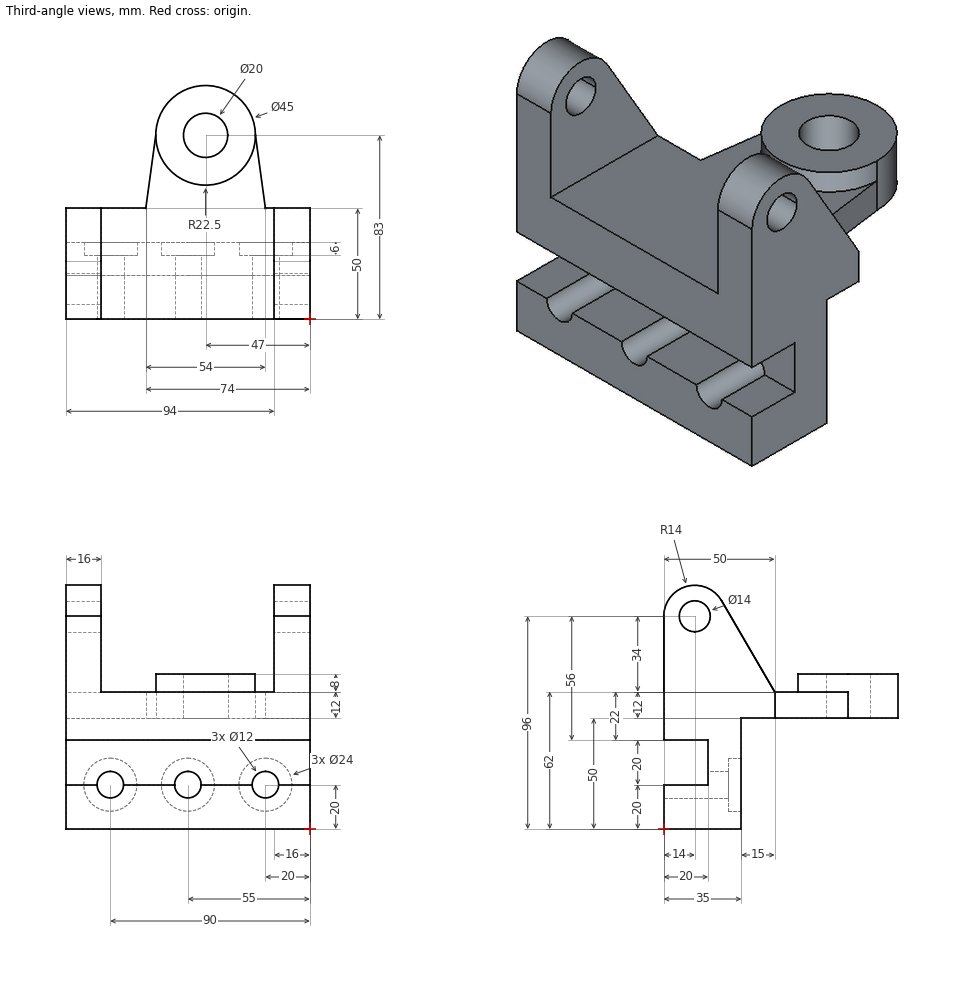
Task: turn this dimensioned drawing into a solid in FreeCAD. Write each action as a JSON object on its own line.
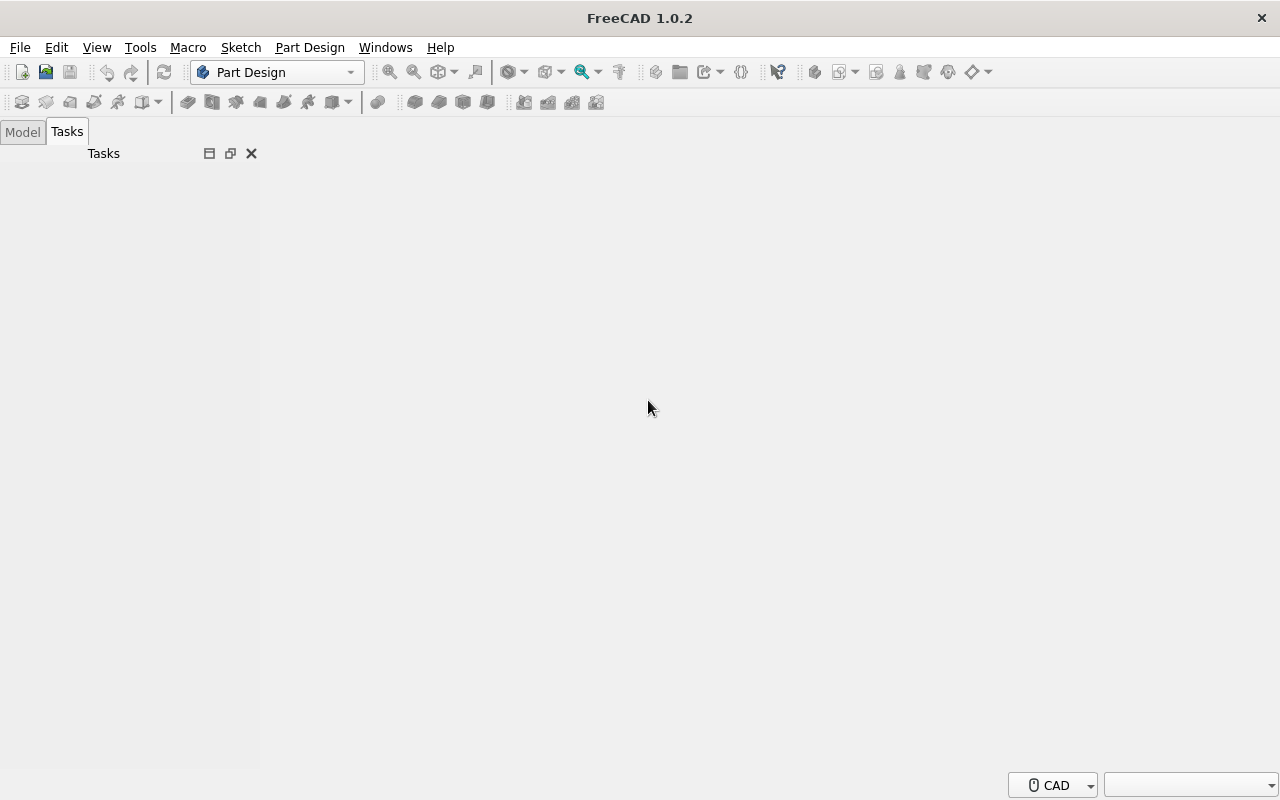
{"action": "key", "text": "ctrl+n"}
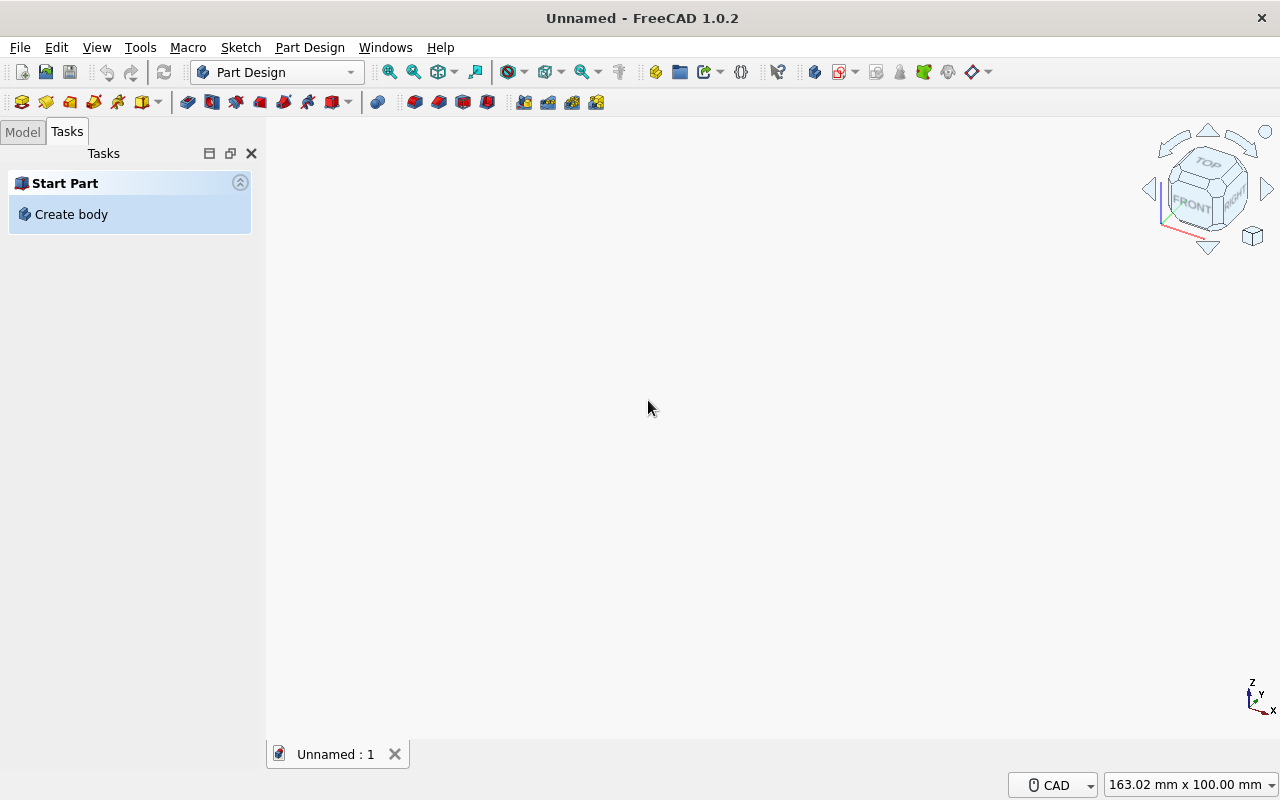
{"action": "left_click", "coordinate": [840, 72]}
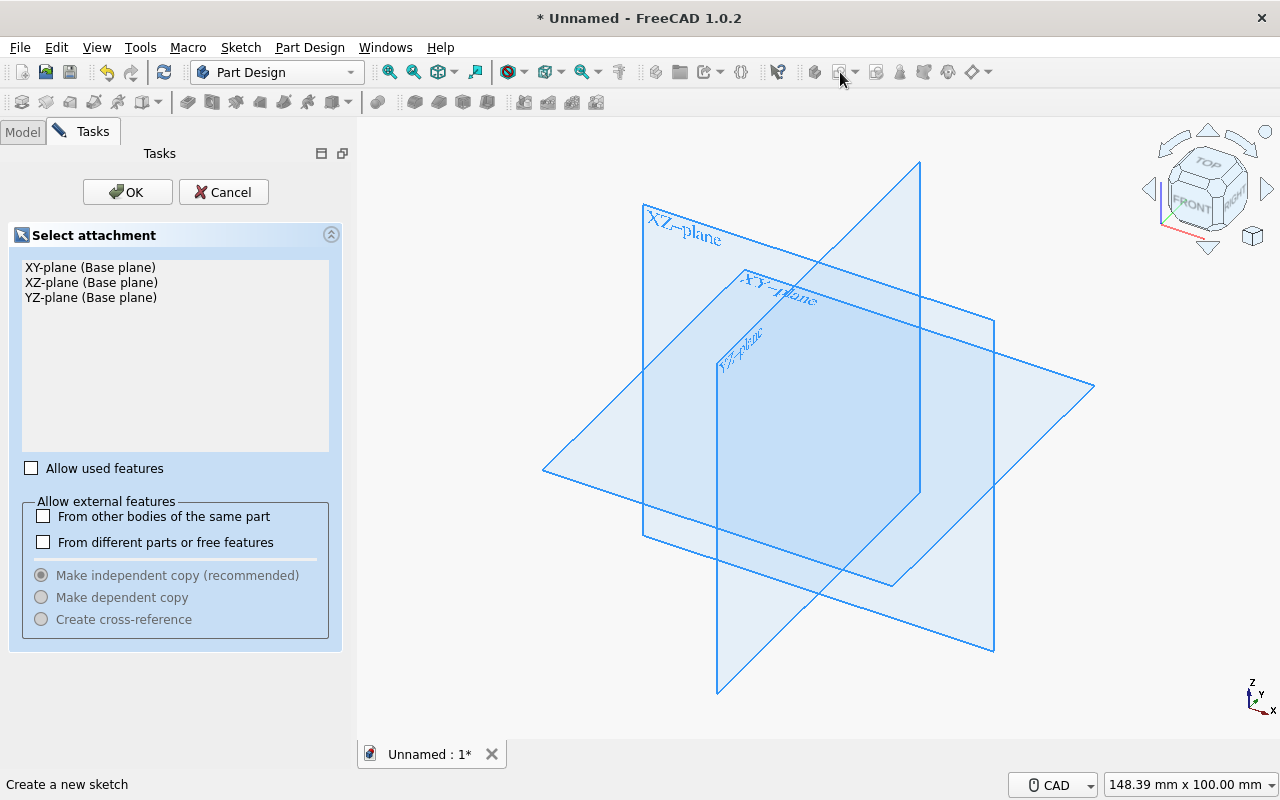
{"action": "left_click", "coordinate": [82, 298]}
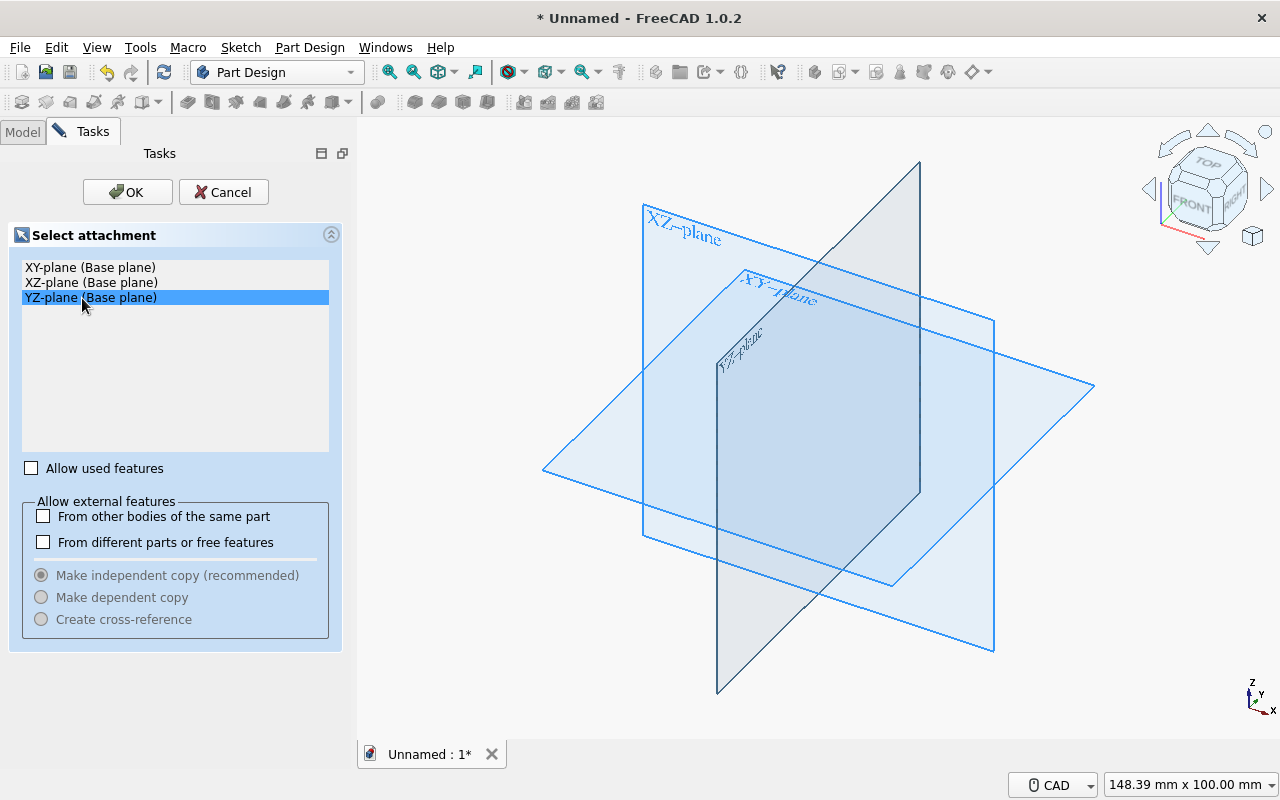
{"action": "left_click", "coordinate": [128, 192]}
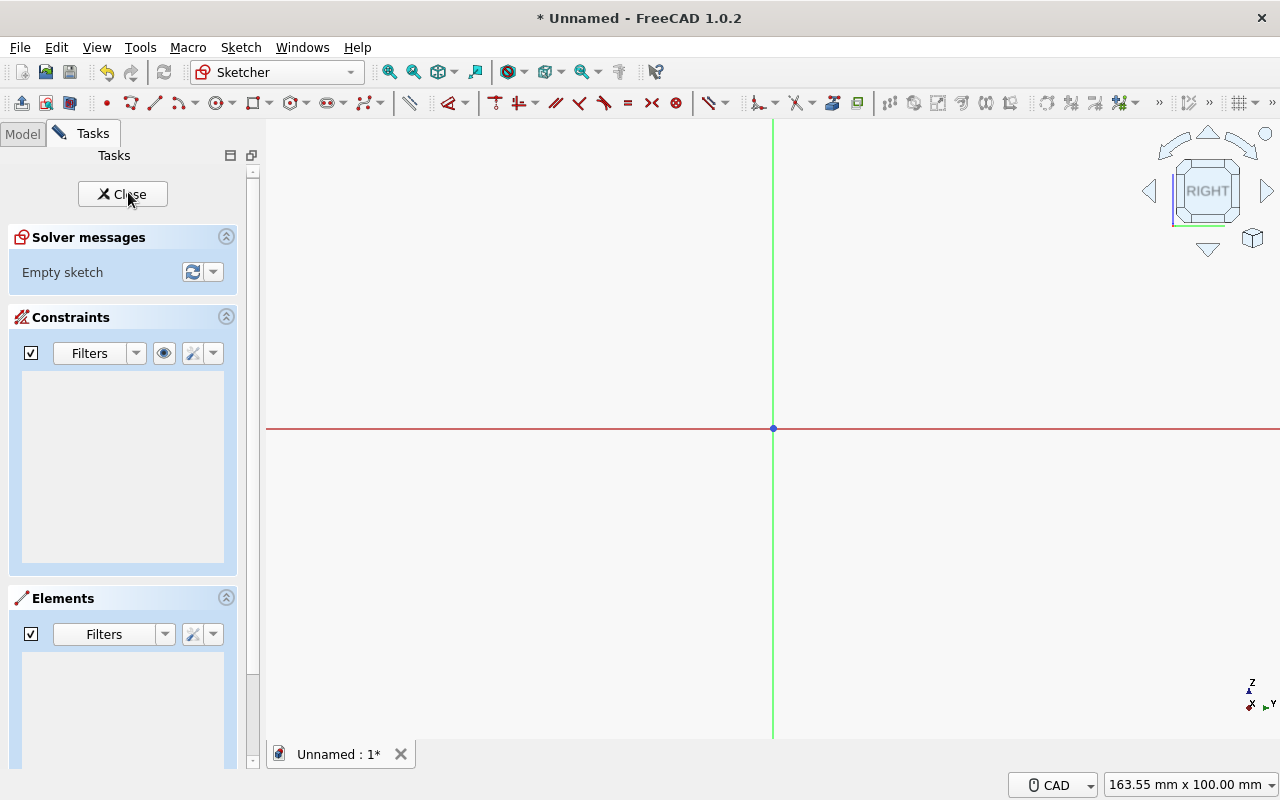
{"action": "scroll", "coordinate": [433, 711], "scroll_direction": "down", "scroll_amount": 3}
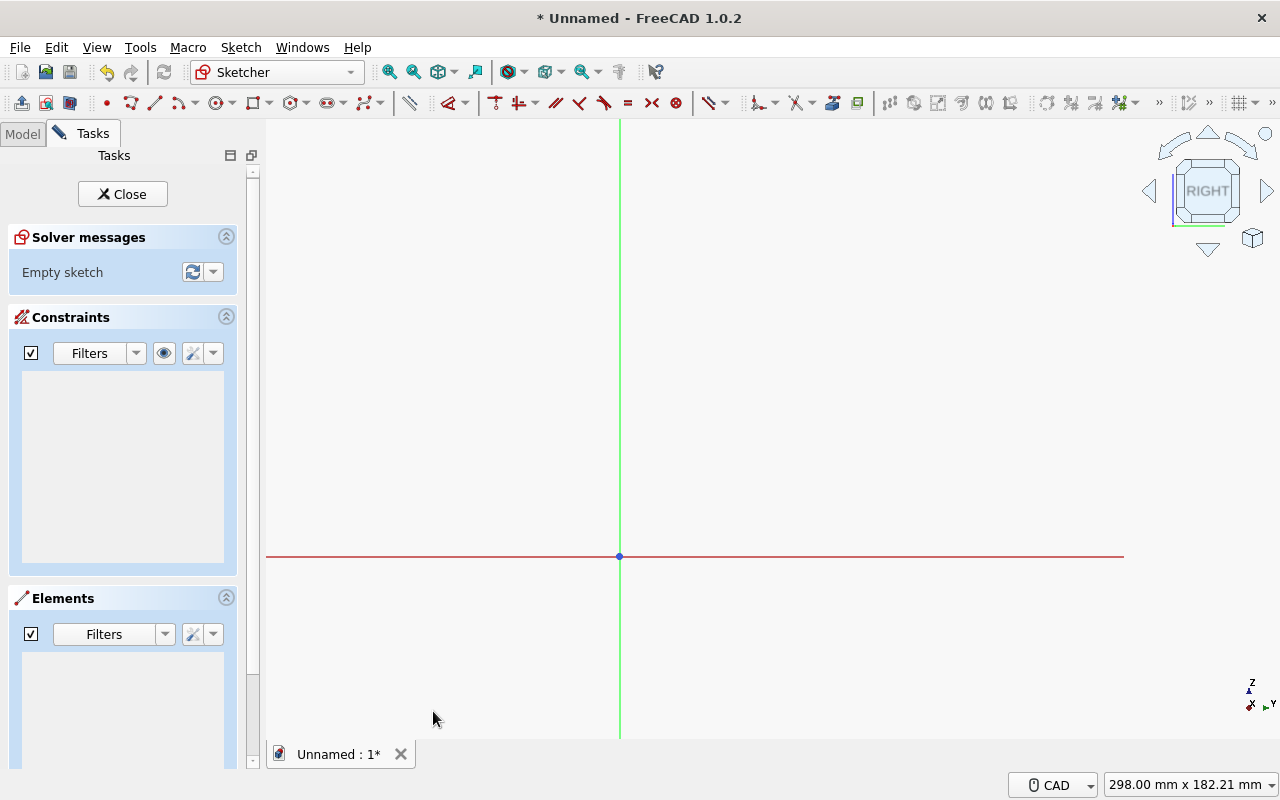
{"action": "left_click", "coordinate": [132, 104]}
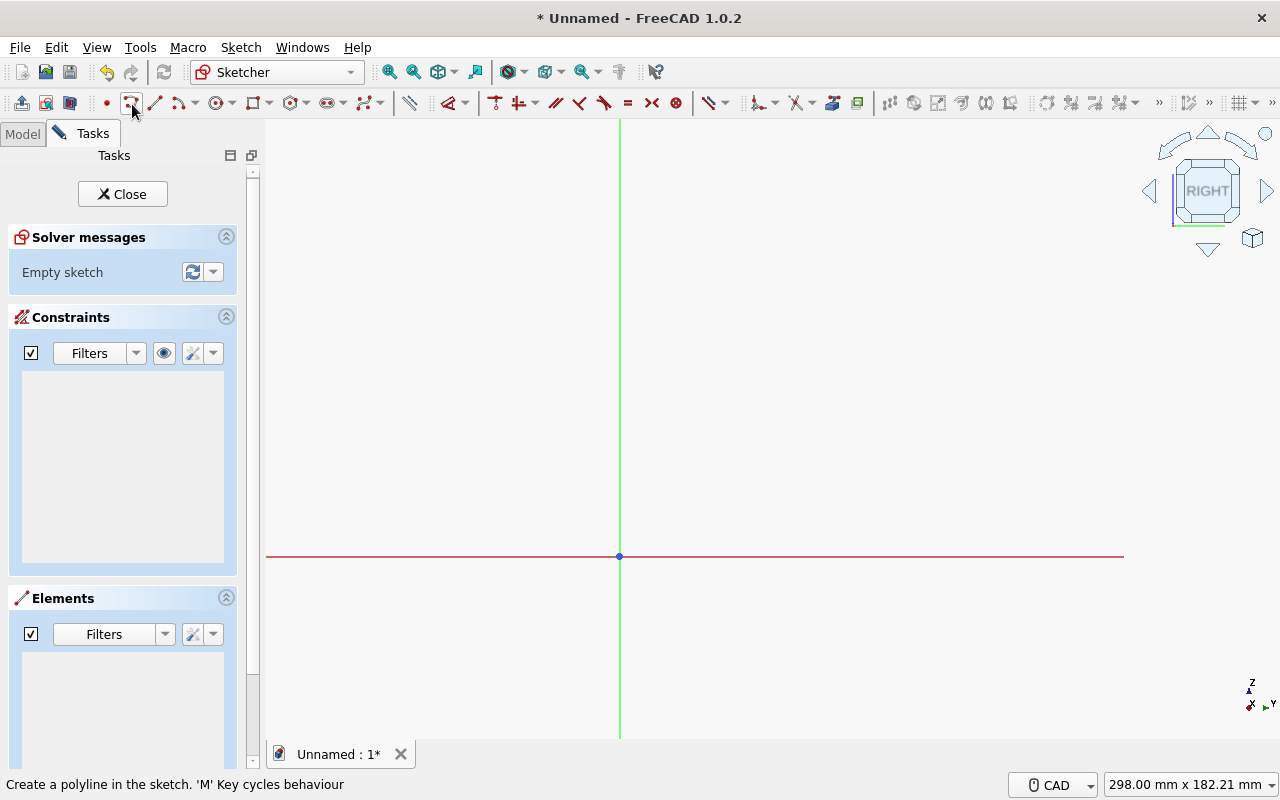
{"action": "left_click", "coordinate": [620, 230]}
{"action": "left_click", "coordinate": [629, 421]}
{"action": "left_click", "coordinate": [688, 421]}
{"action": "left_click", "coordinate": [688, 489]}
{"action": "left_click", "coordinate": [620, 489]}
{"action": "left_click", "coordinate": [620, 557]}
{"action": "left_click", "coordinate": [739, 548]}
{"action": "left_click", "coordinate": [739, 387]}
{"action": "left_click", "coordinate": [790, 387]}
{"action": "left_click", "coordinate": [790, 346]}
{"action": "left_click", "coordinate": [708, 206]}
{"action": "right_click", "coordinate": [708, 206]}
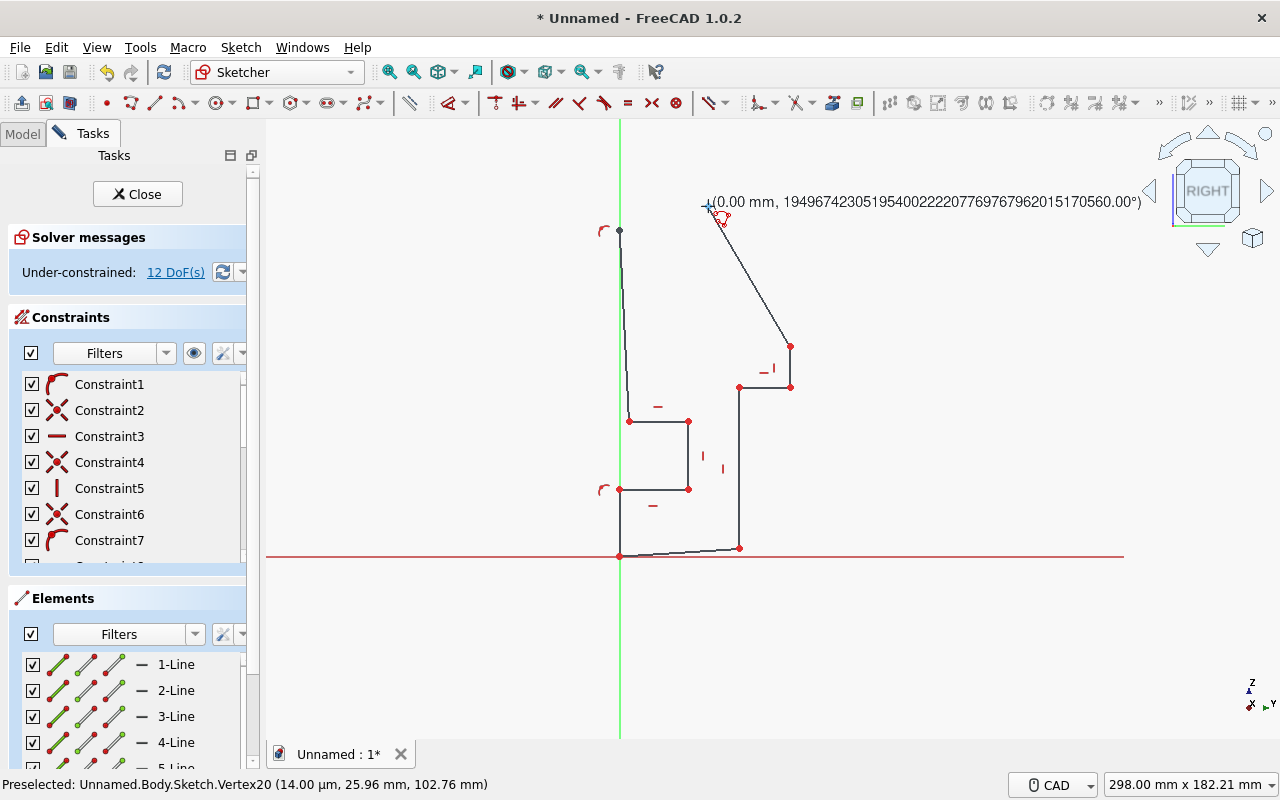
{"action": "left_click", "coordinate": [198, 104]}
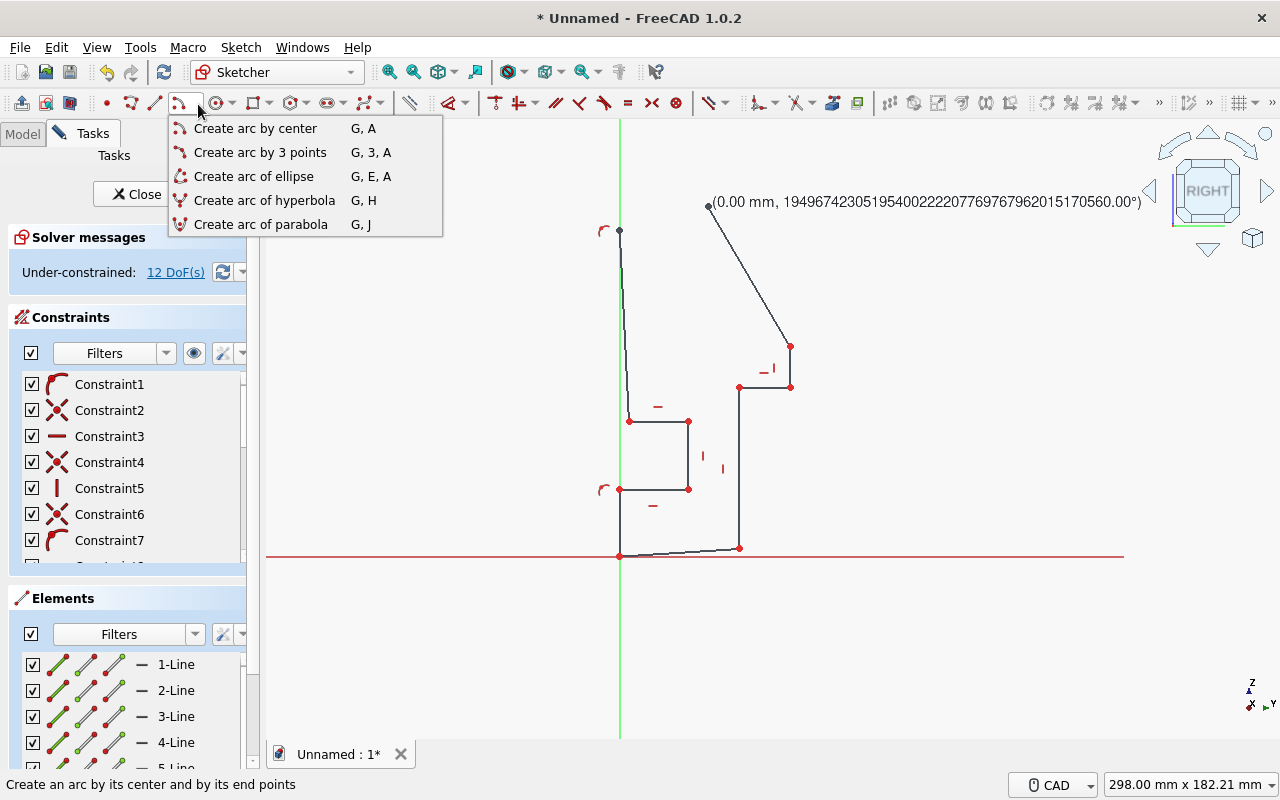
{"action": "left_click", "coordinate": [306, 152]}